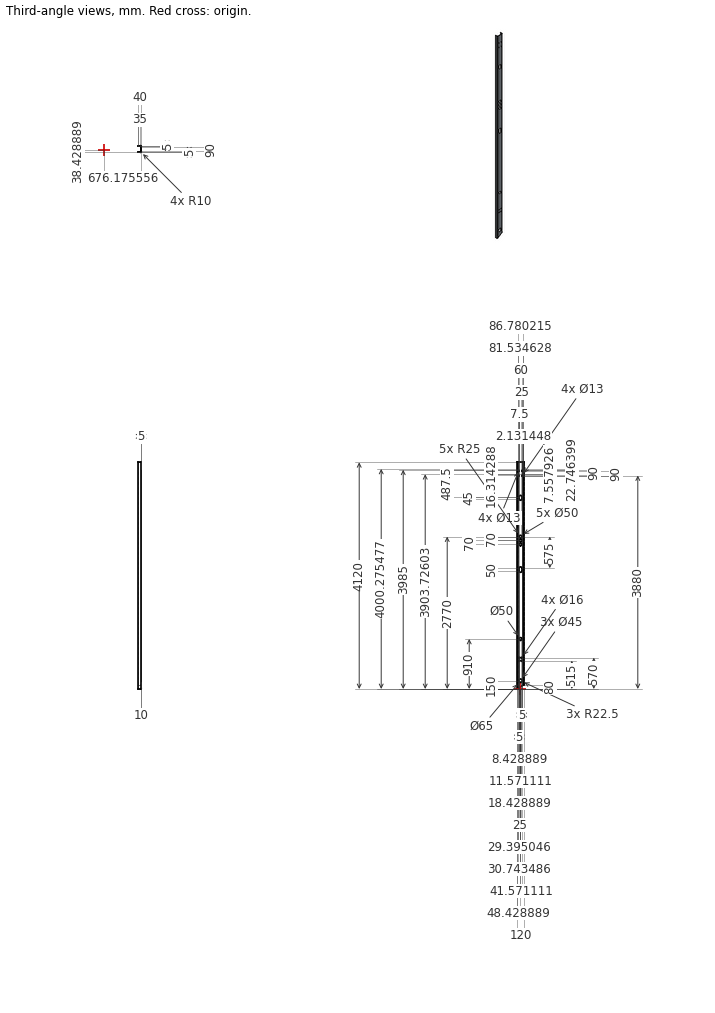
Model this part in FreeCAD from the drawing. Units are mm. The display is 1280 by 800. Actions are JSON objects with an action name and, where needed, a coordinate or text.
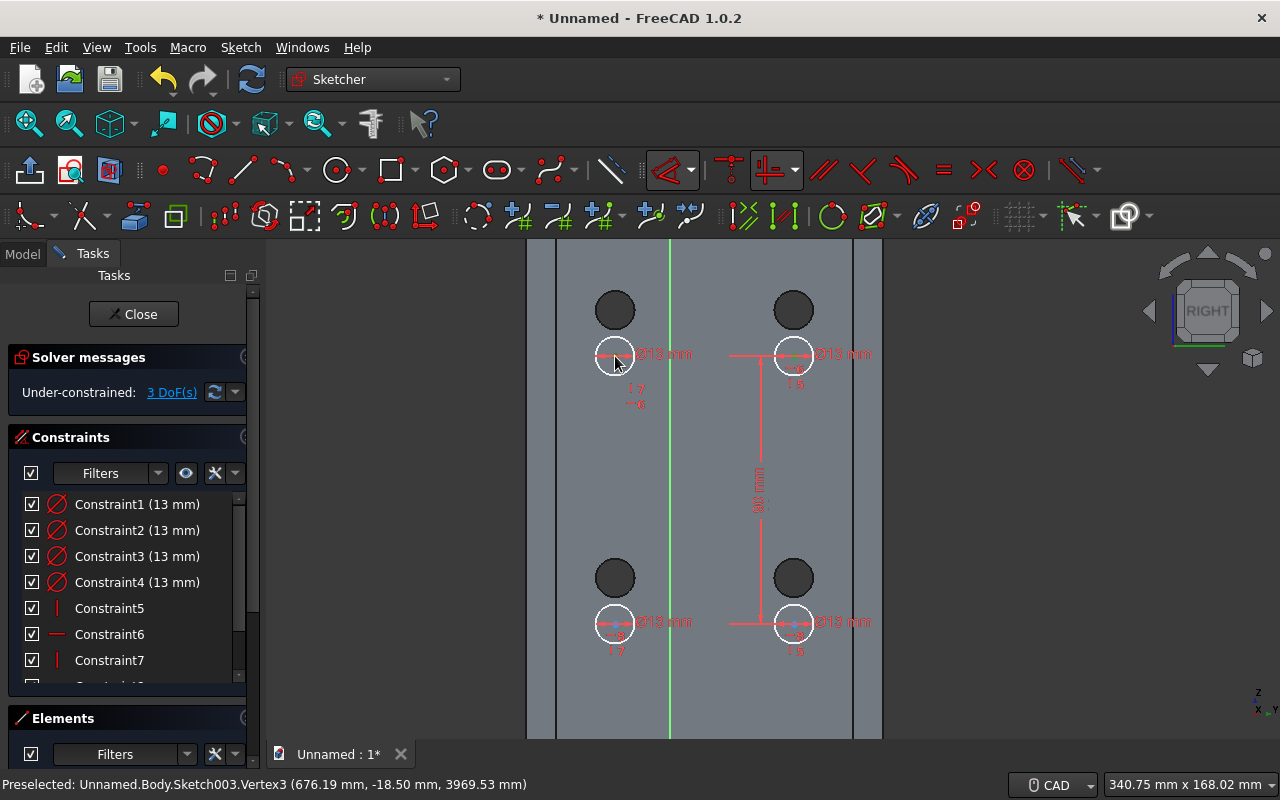
{"action": "left_click", "coordinate": [694, 170]}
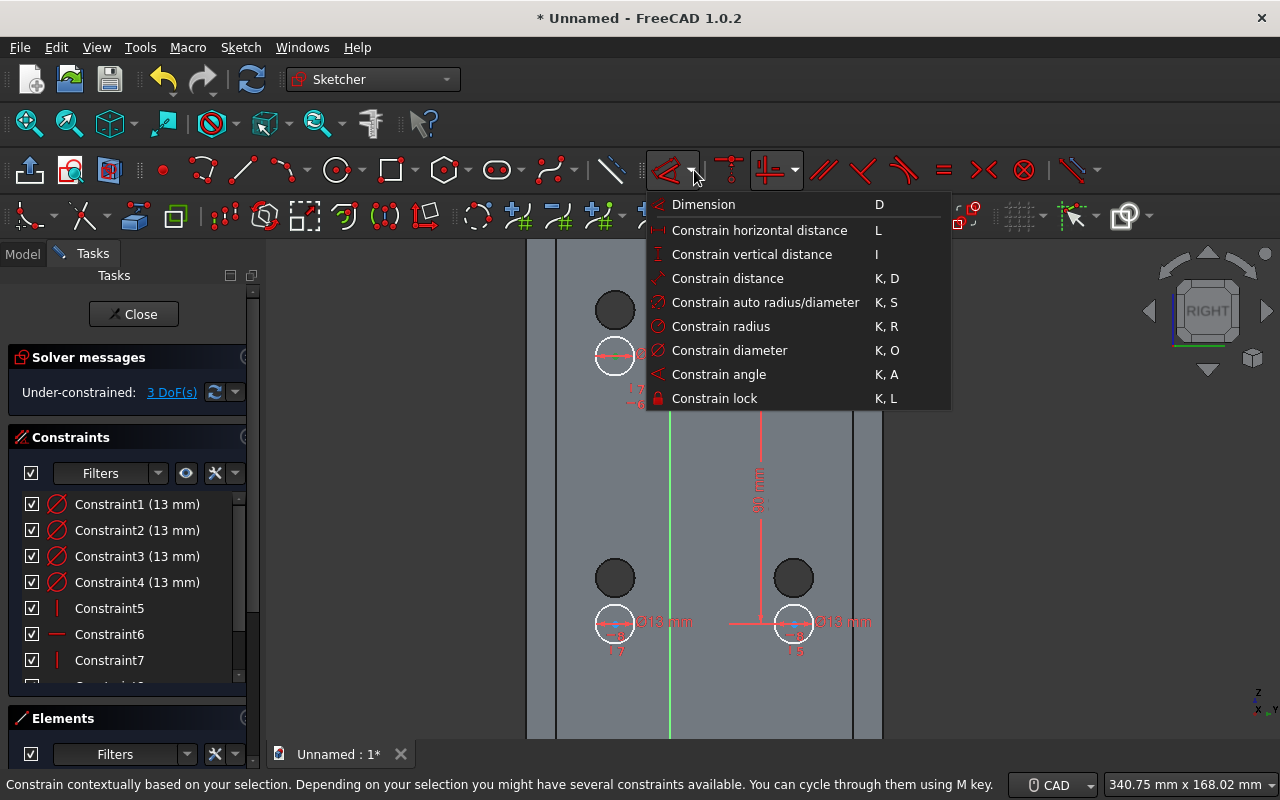
{"action": "left_click", "coordinate": [799, 230]}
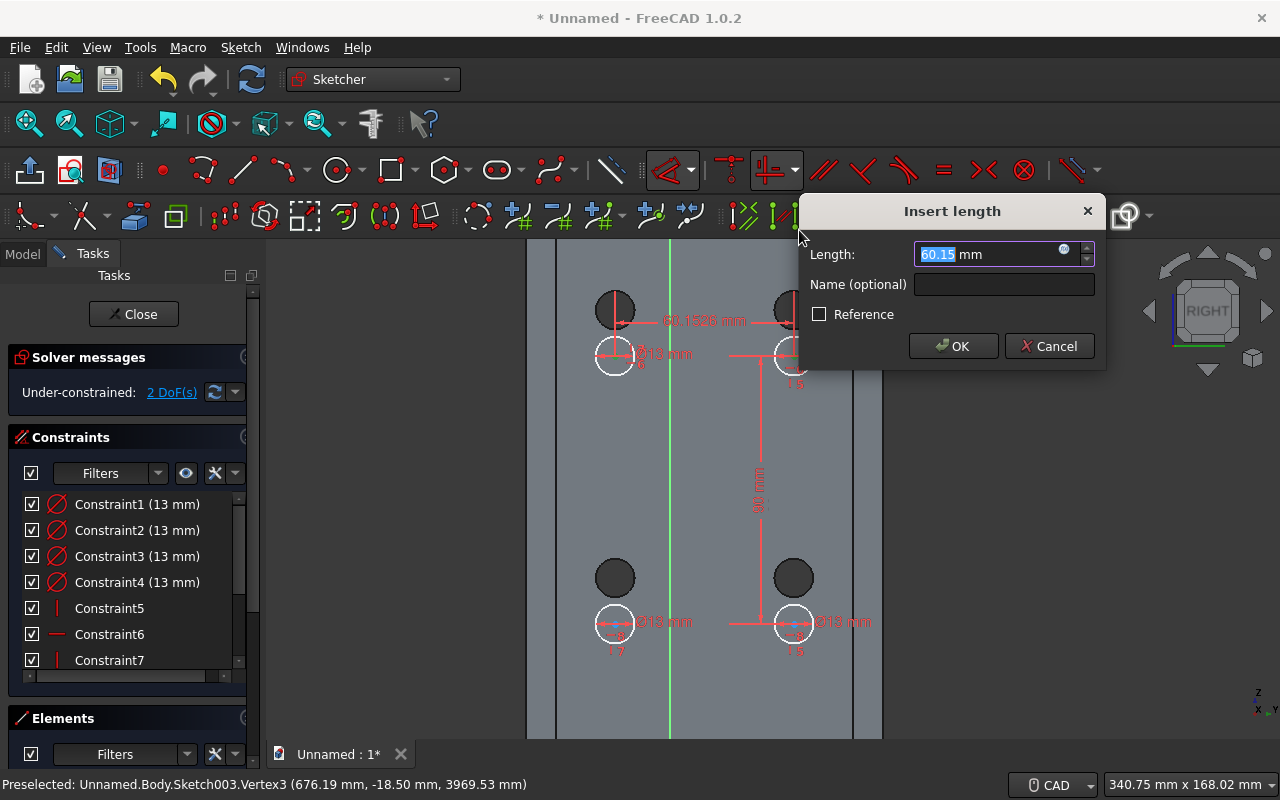
{"action": "type", "text": "60"}
{"action": "key", "text": "Return"}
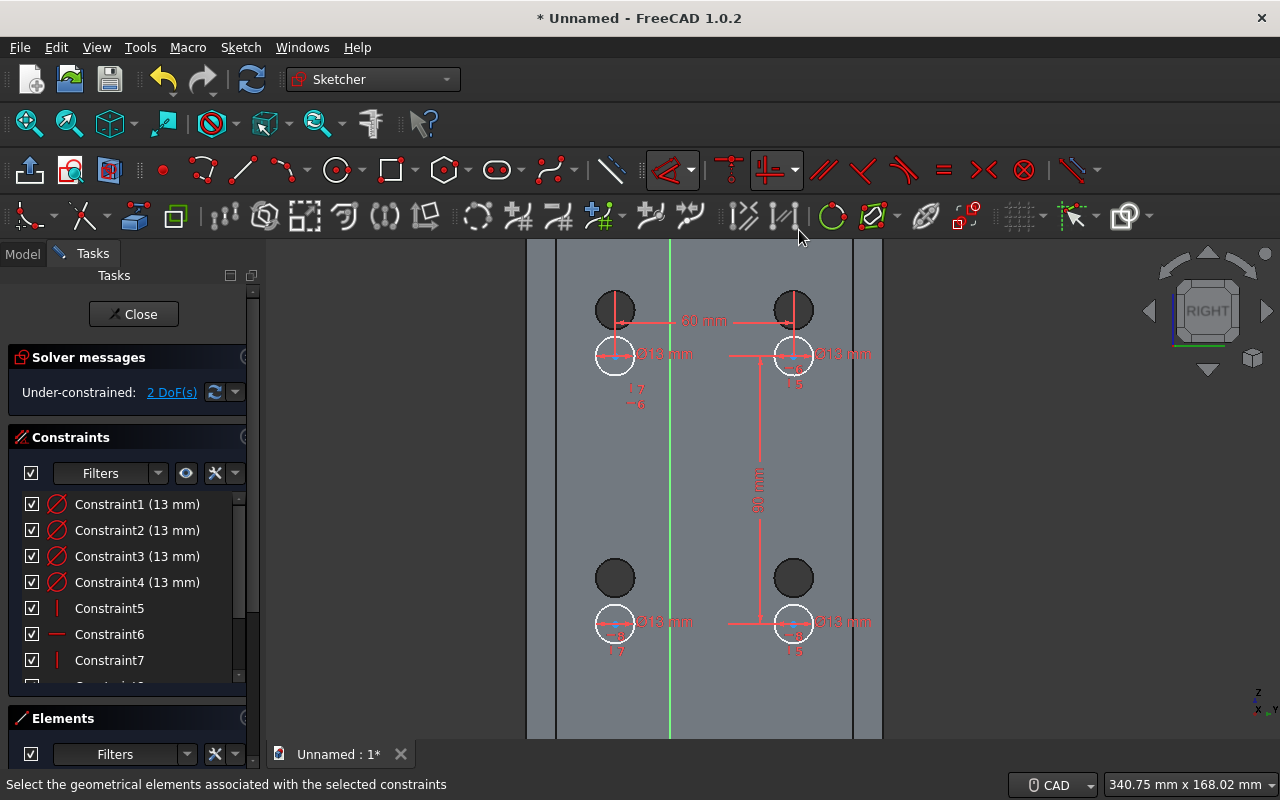
{"action": "left_click", "coordinate": [794, 624]}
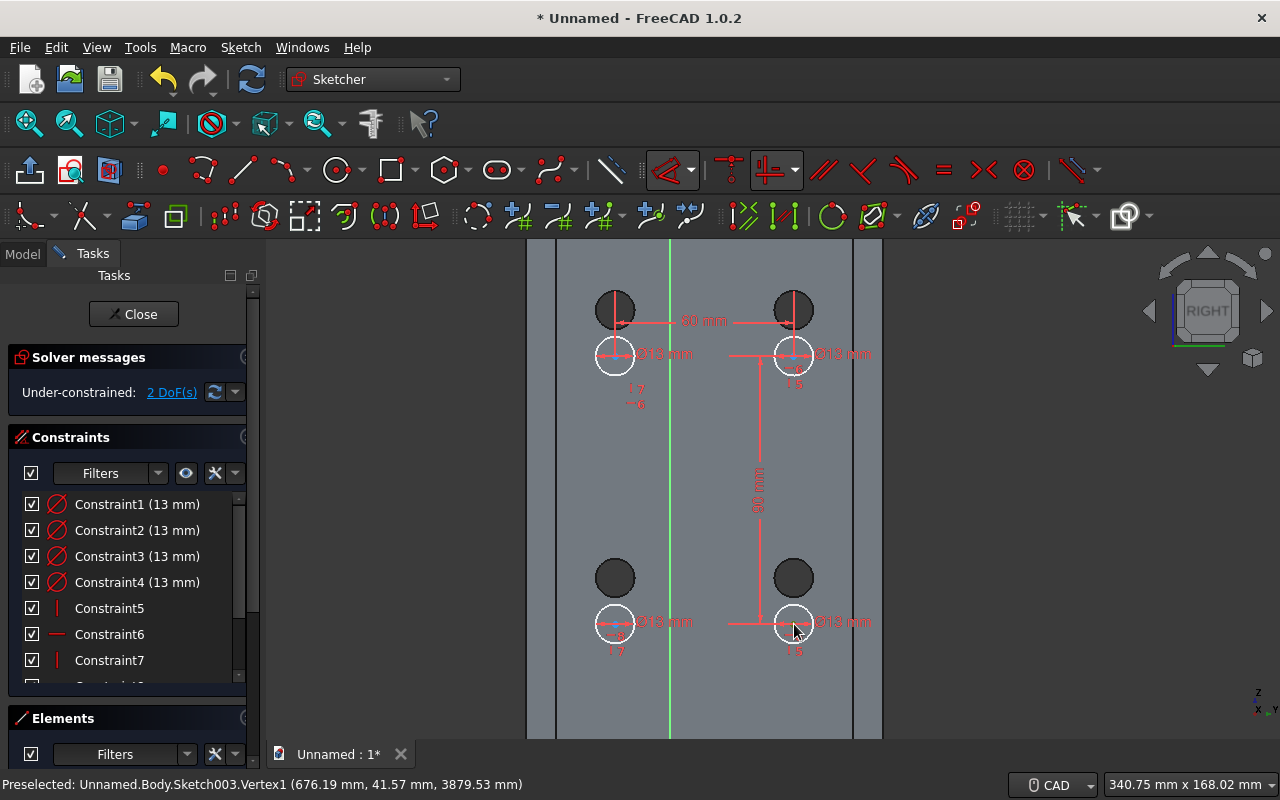
{"action": "key", "text": "i"}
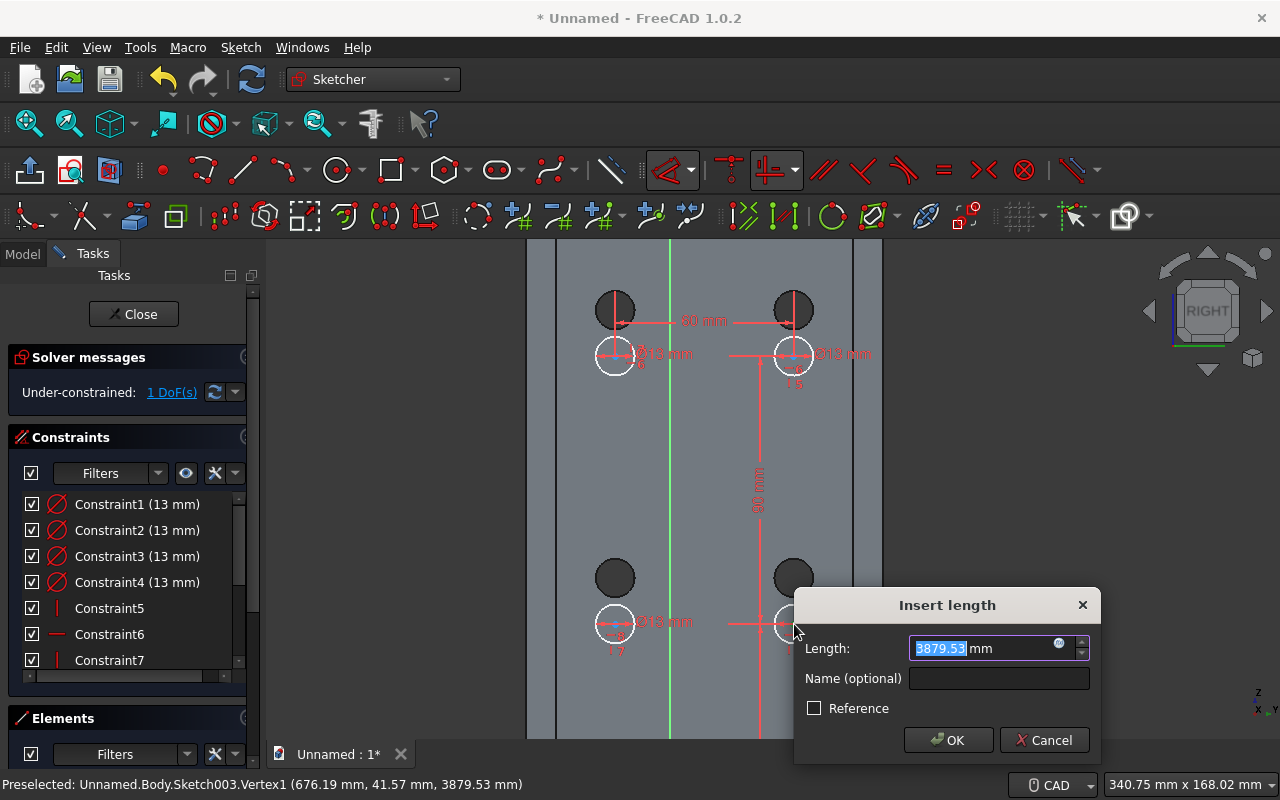
{"action": "type", "text": "3880"}
{"action": "key", "text": "Return"}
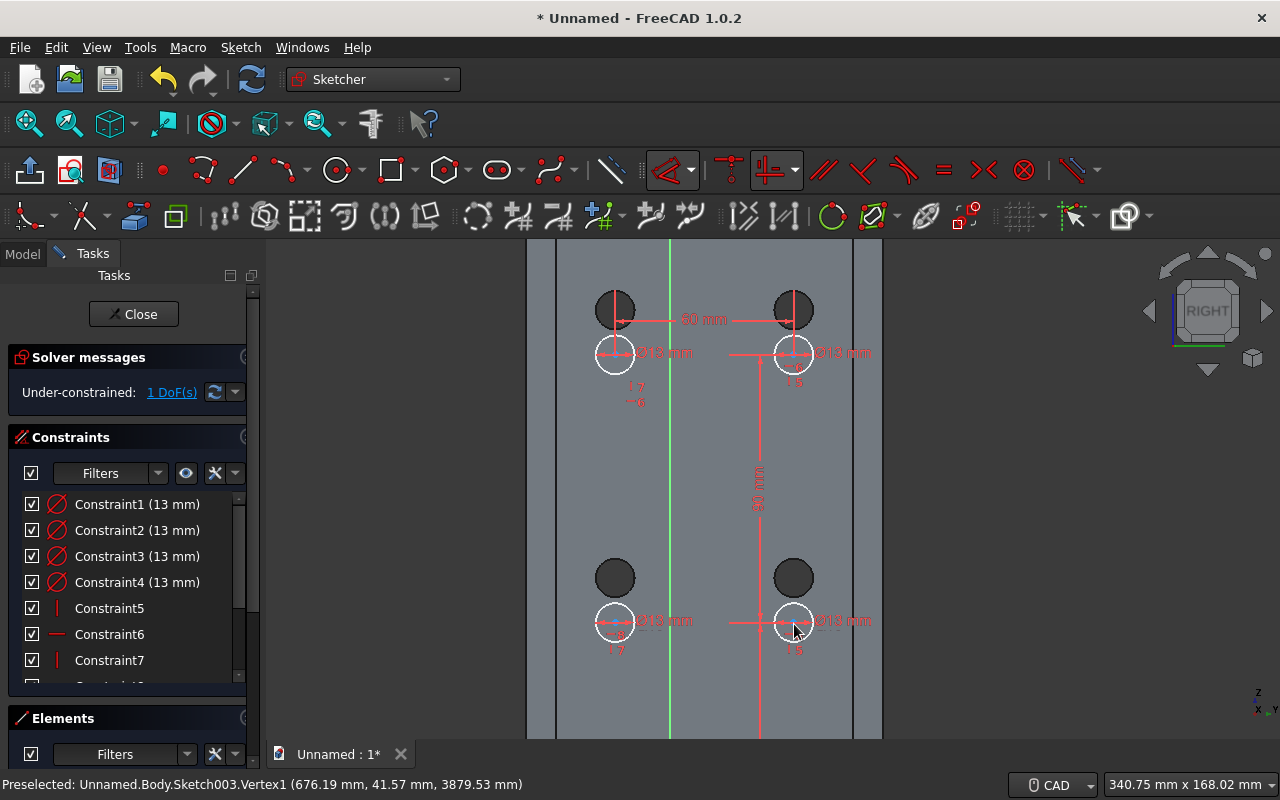
{"action": "left_click", "coordinate": [794, 623]}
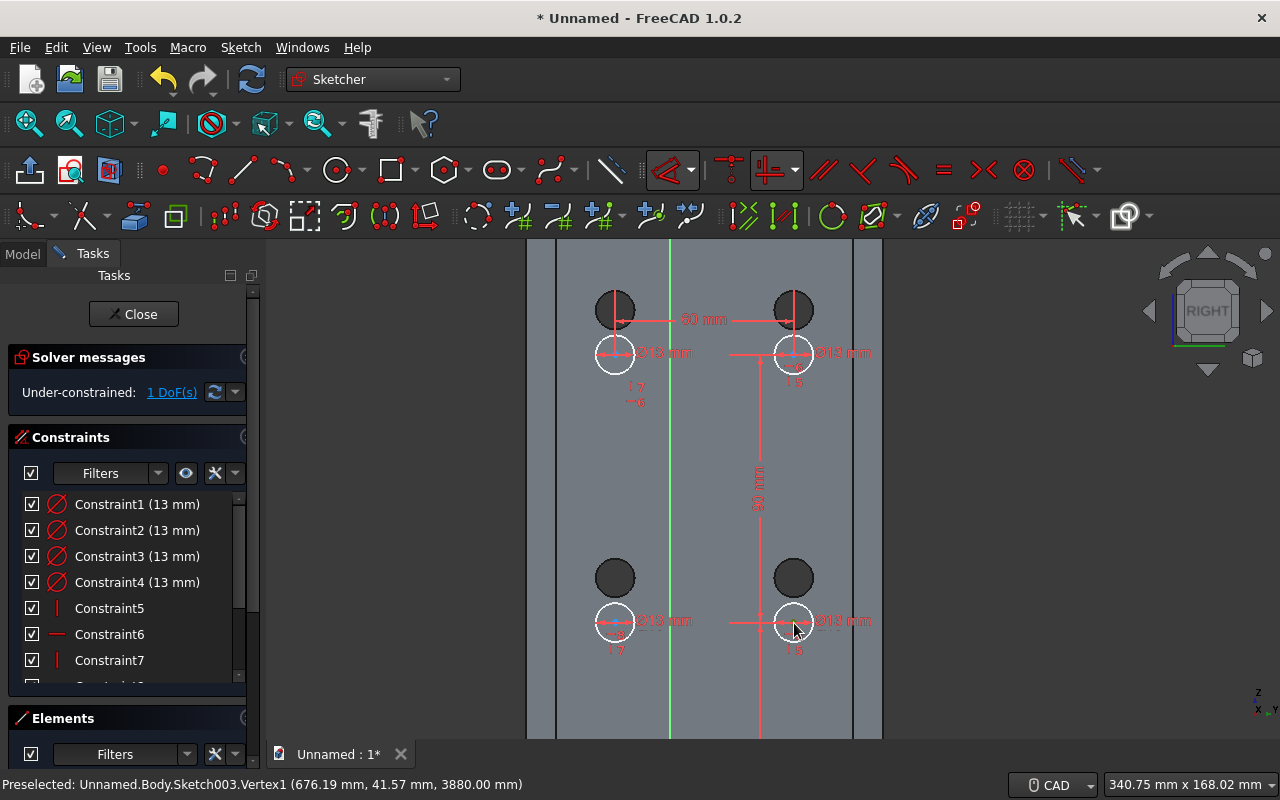
{"action": "key", "text": "l"}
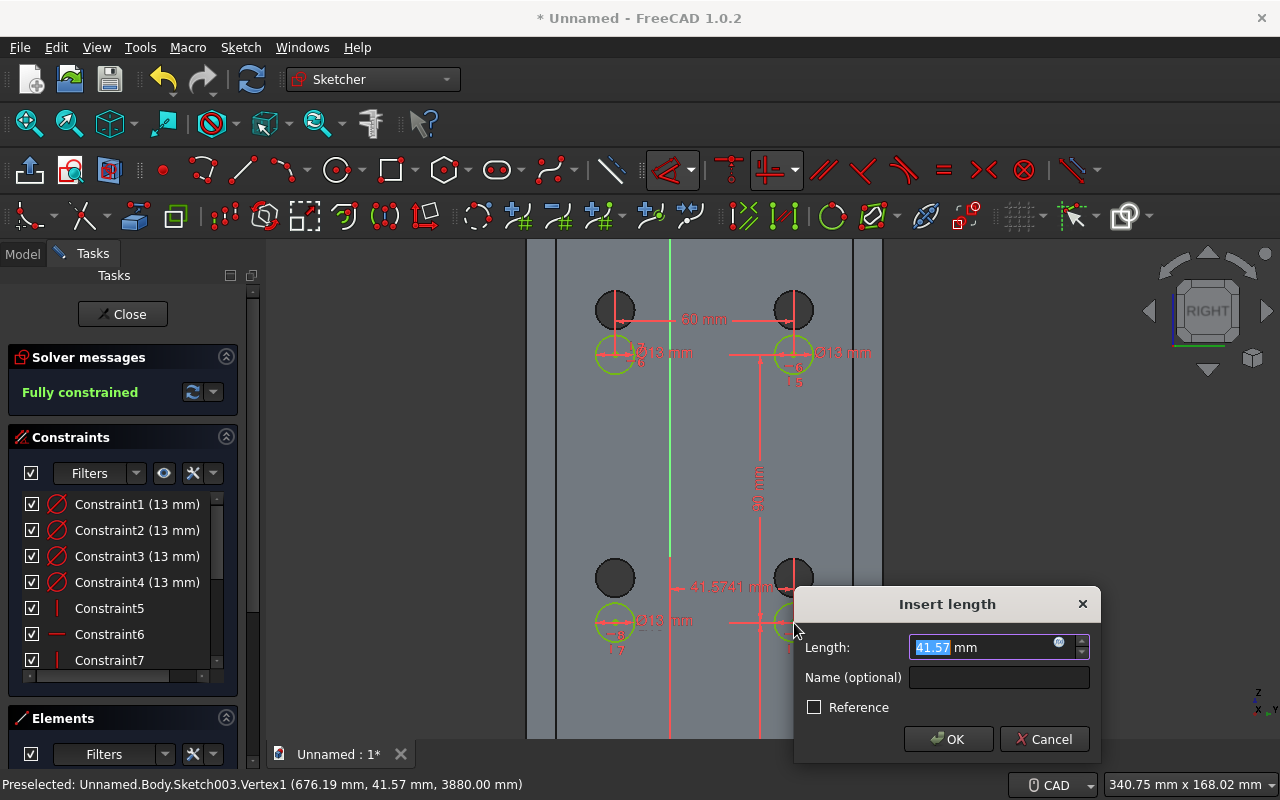
{"action": "type", "text": "41.571111"}
{"action": "key", "text": "Return"}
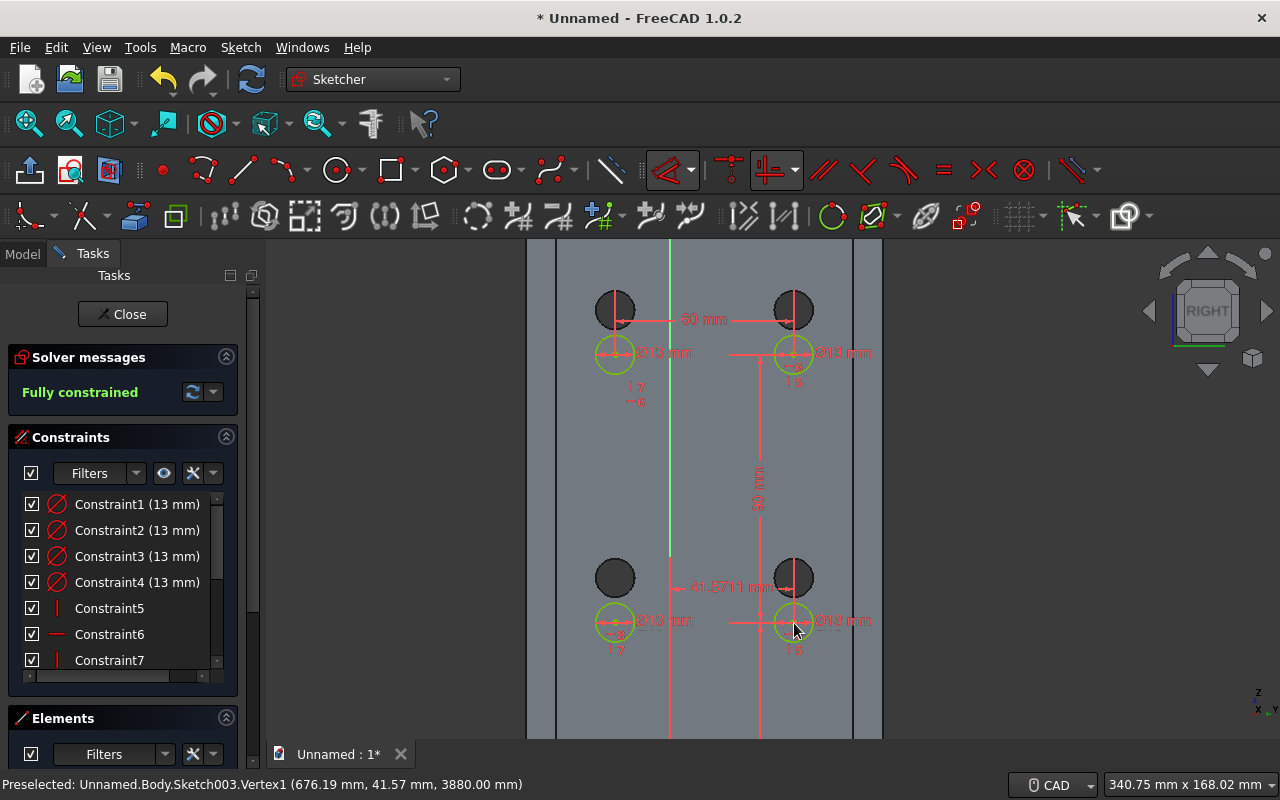
{"action": "left_click", "coordinate": [123, 314]}